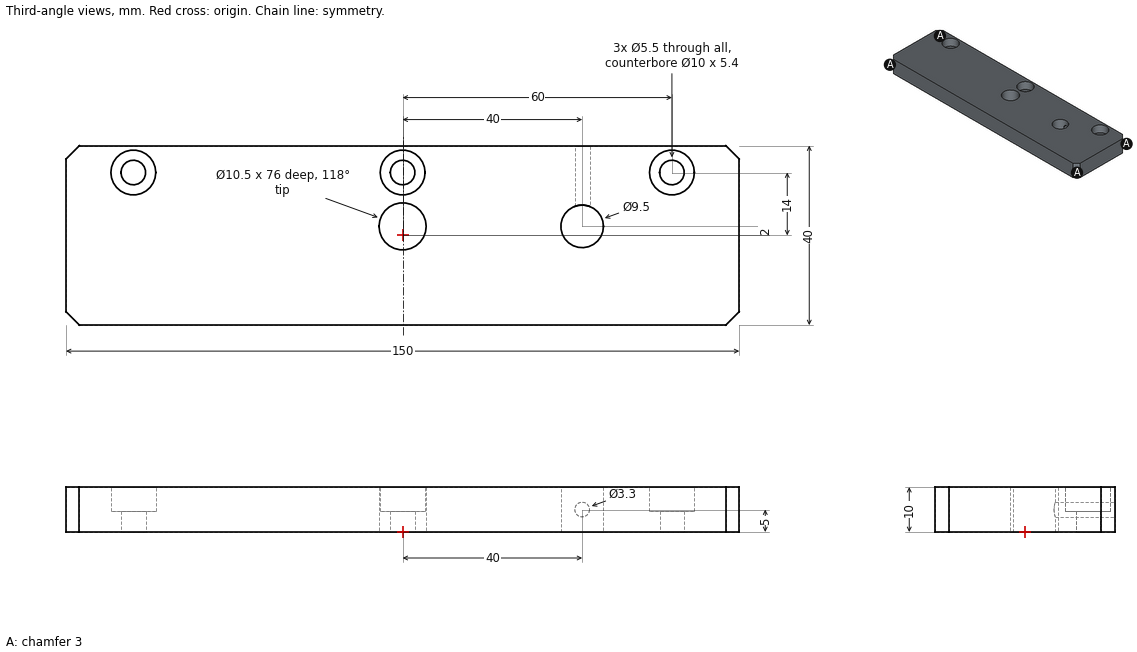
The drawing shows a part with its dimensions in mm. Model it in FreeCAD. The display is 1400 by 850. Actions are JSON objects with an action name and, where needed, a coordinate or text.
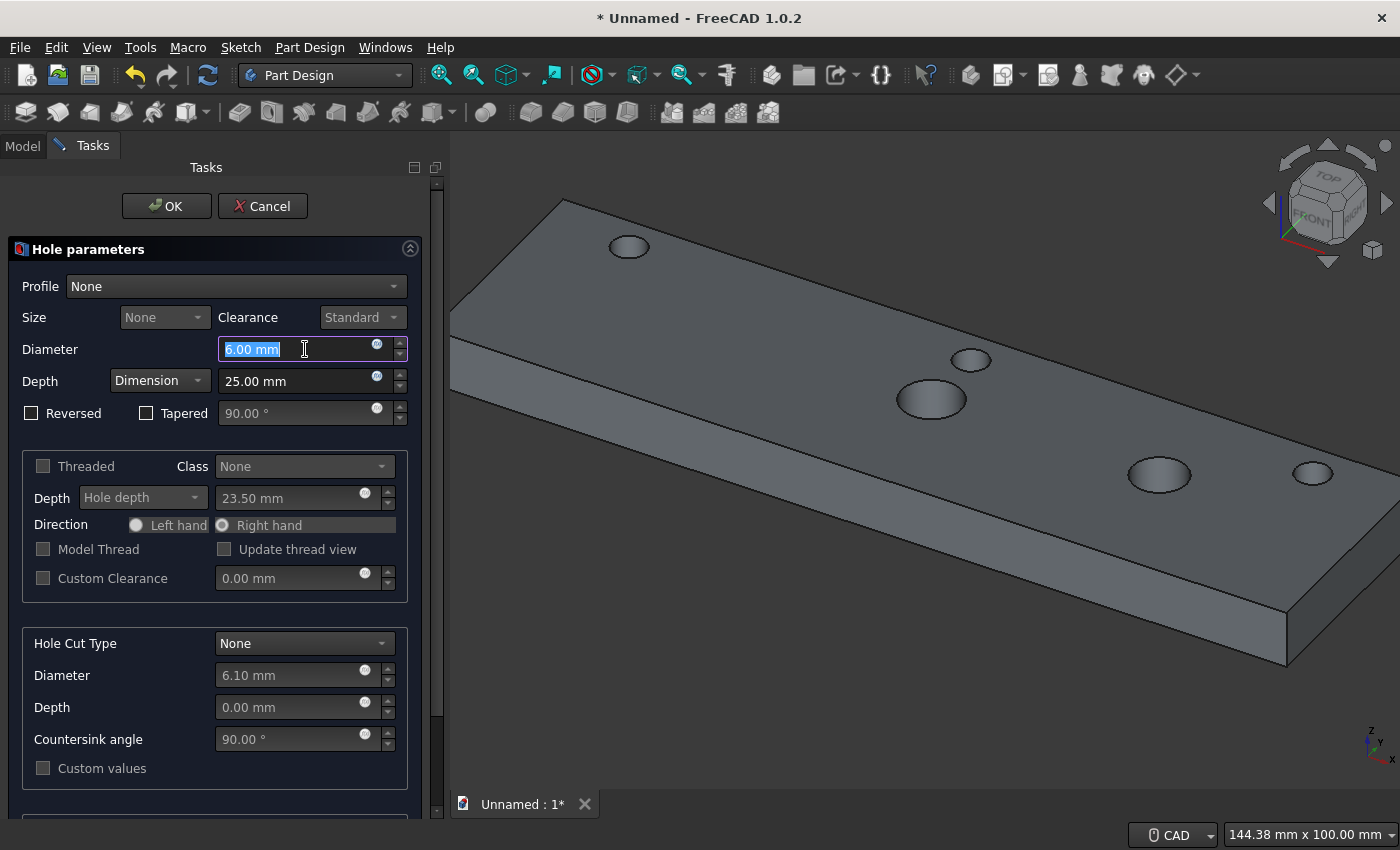
{"action": "type", "text": "5.5"}
{"action": "key", "text": "Tab"}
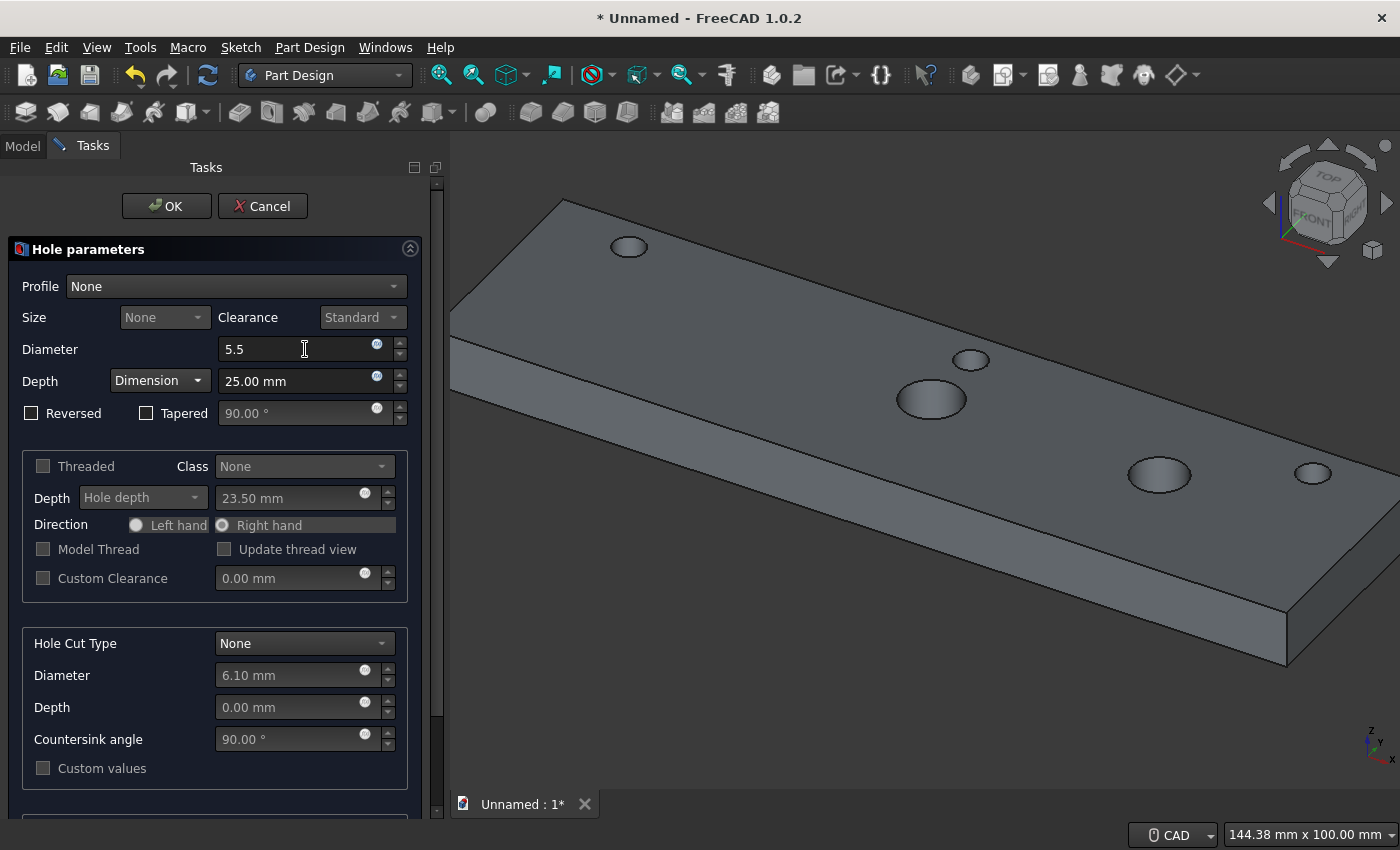
{"action": "left_click", "coordinate": [161, 380]}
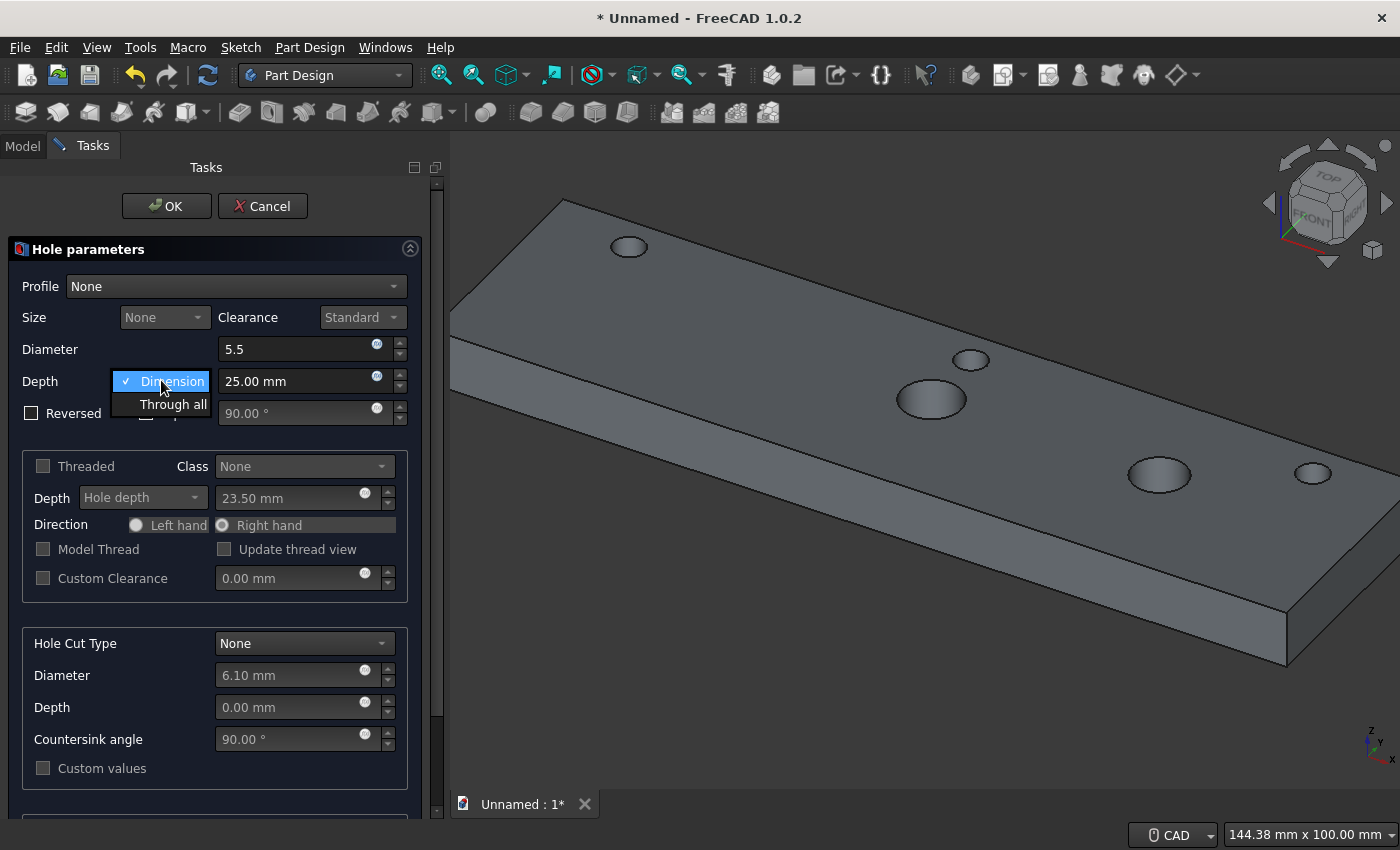
{"action": "left_click", "coordinate": [160, 404]}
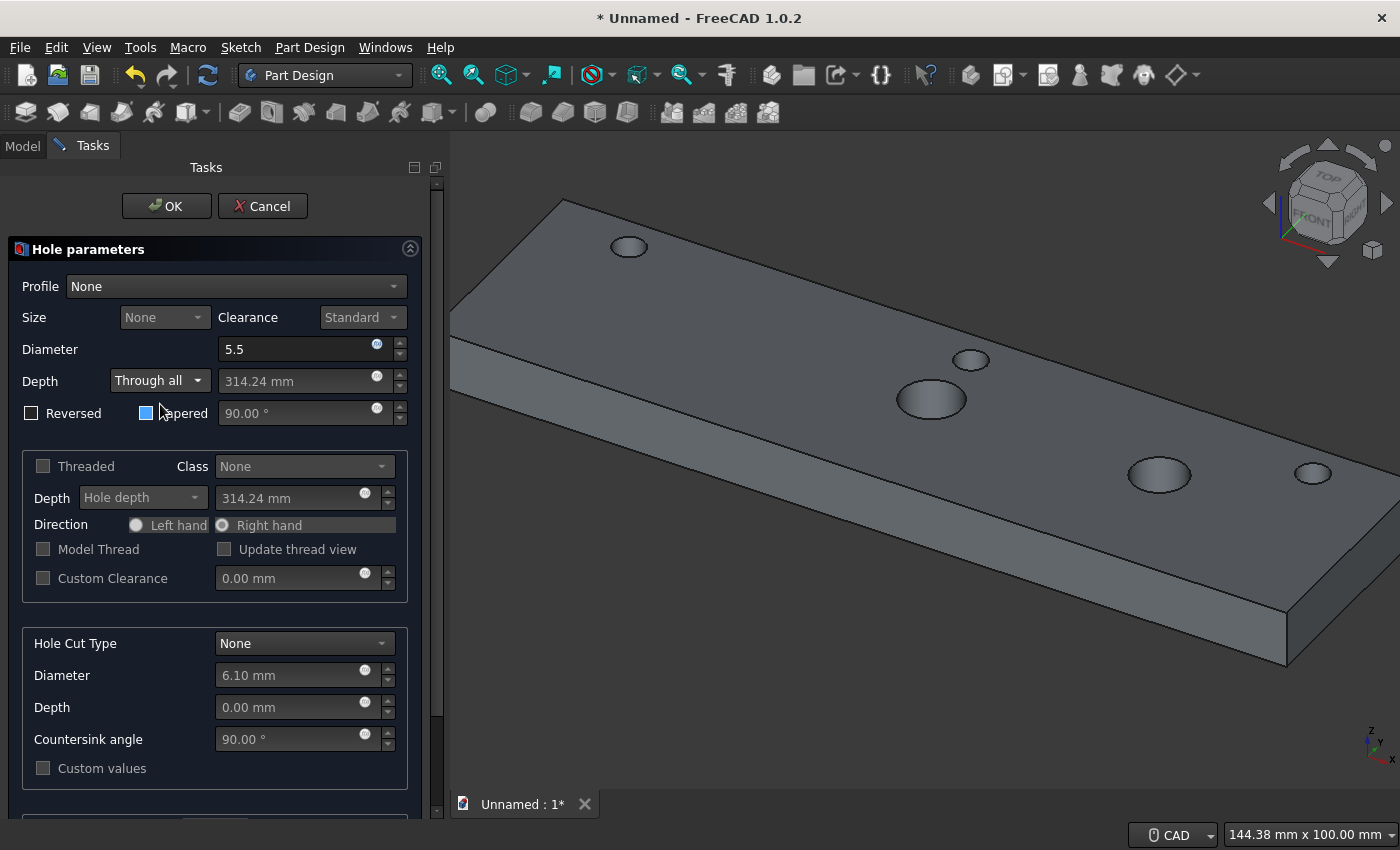
{"action": "left_click", "coordinate": [306, 644]}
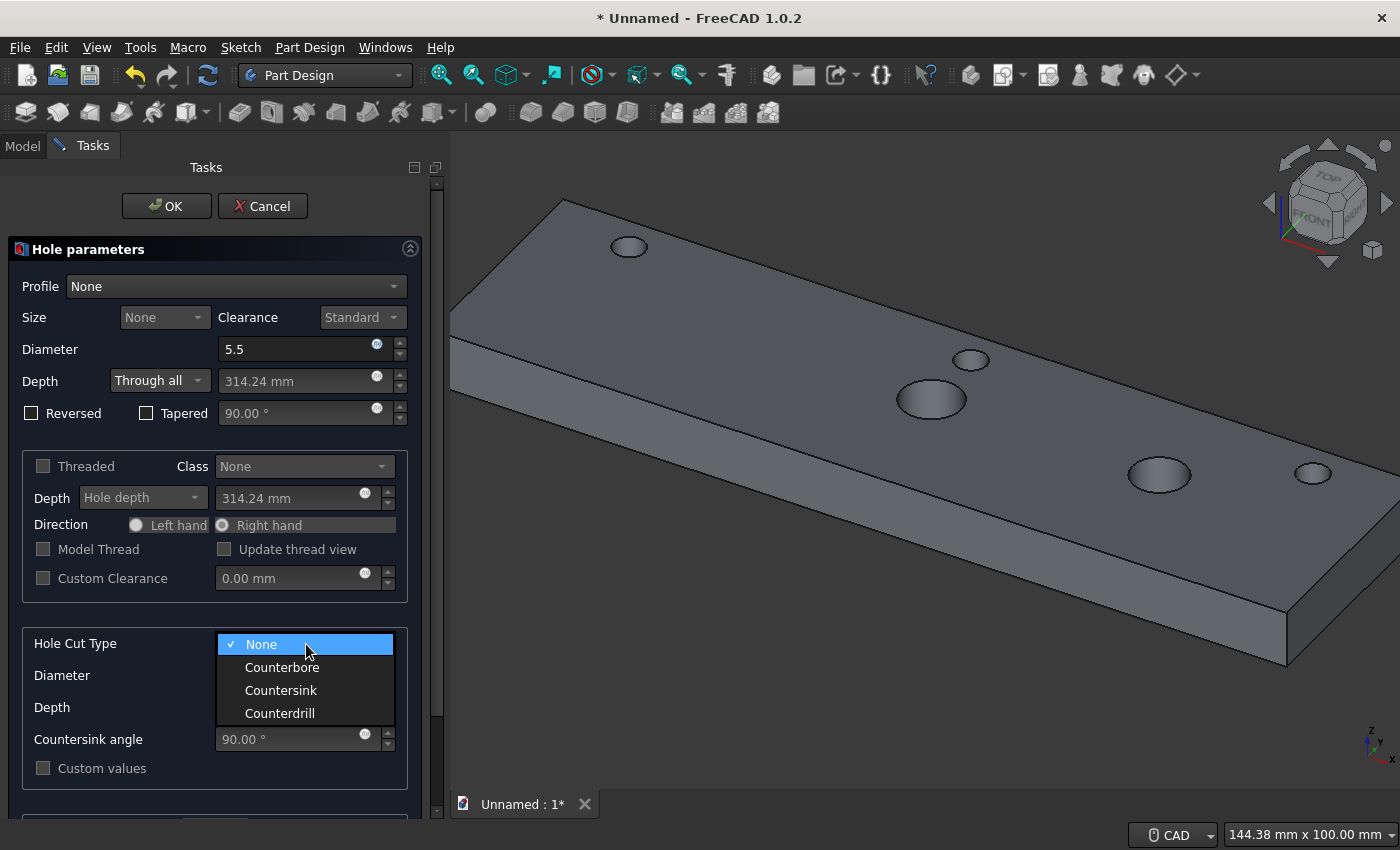
{"action": "left_click", "coordinate": [304, 668]}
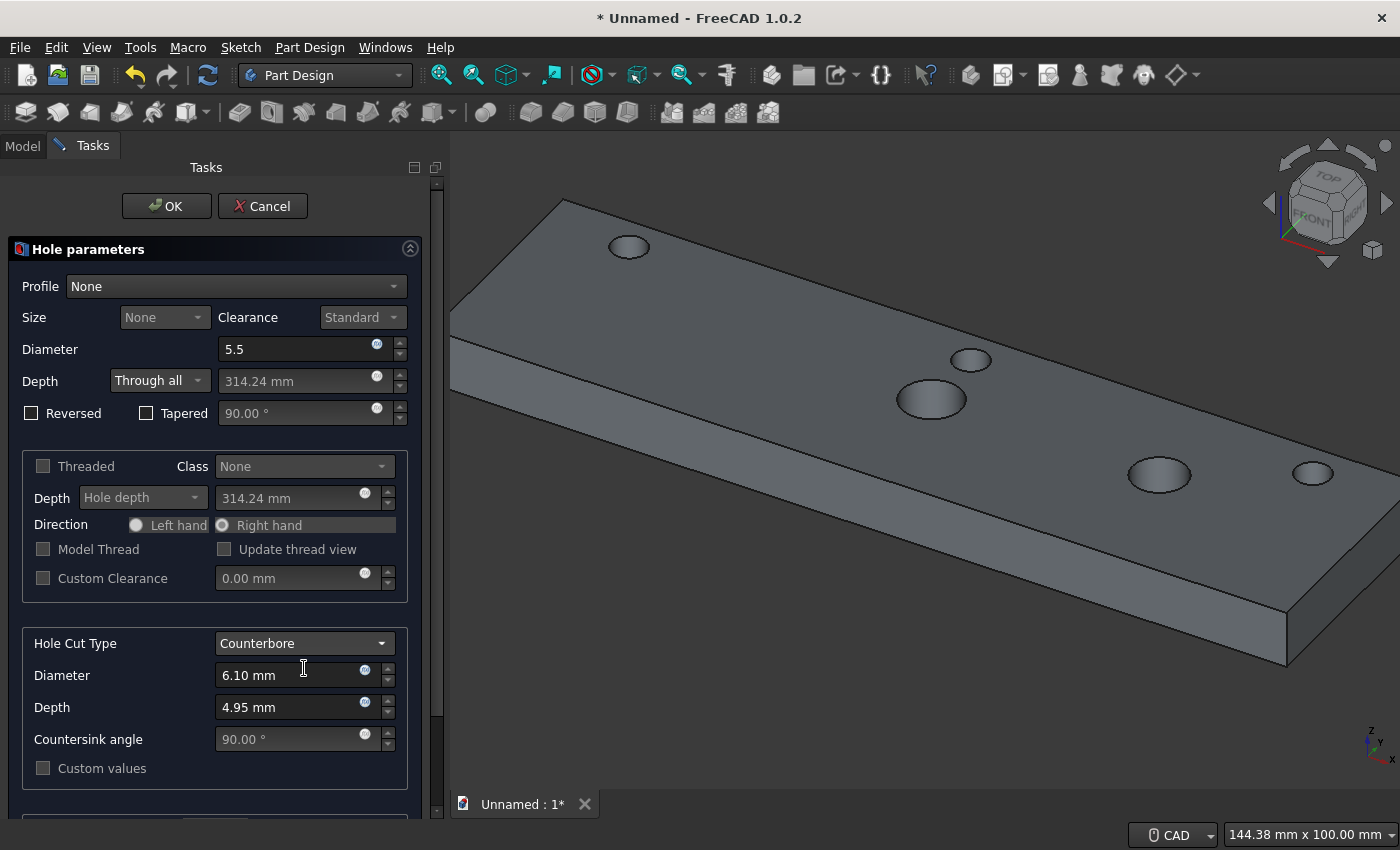
{"action": "triple_click", "coordinate": [298, 675]}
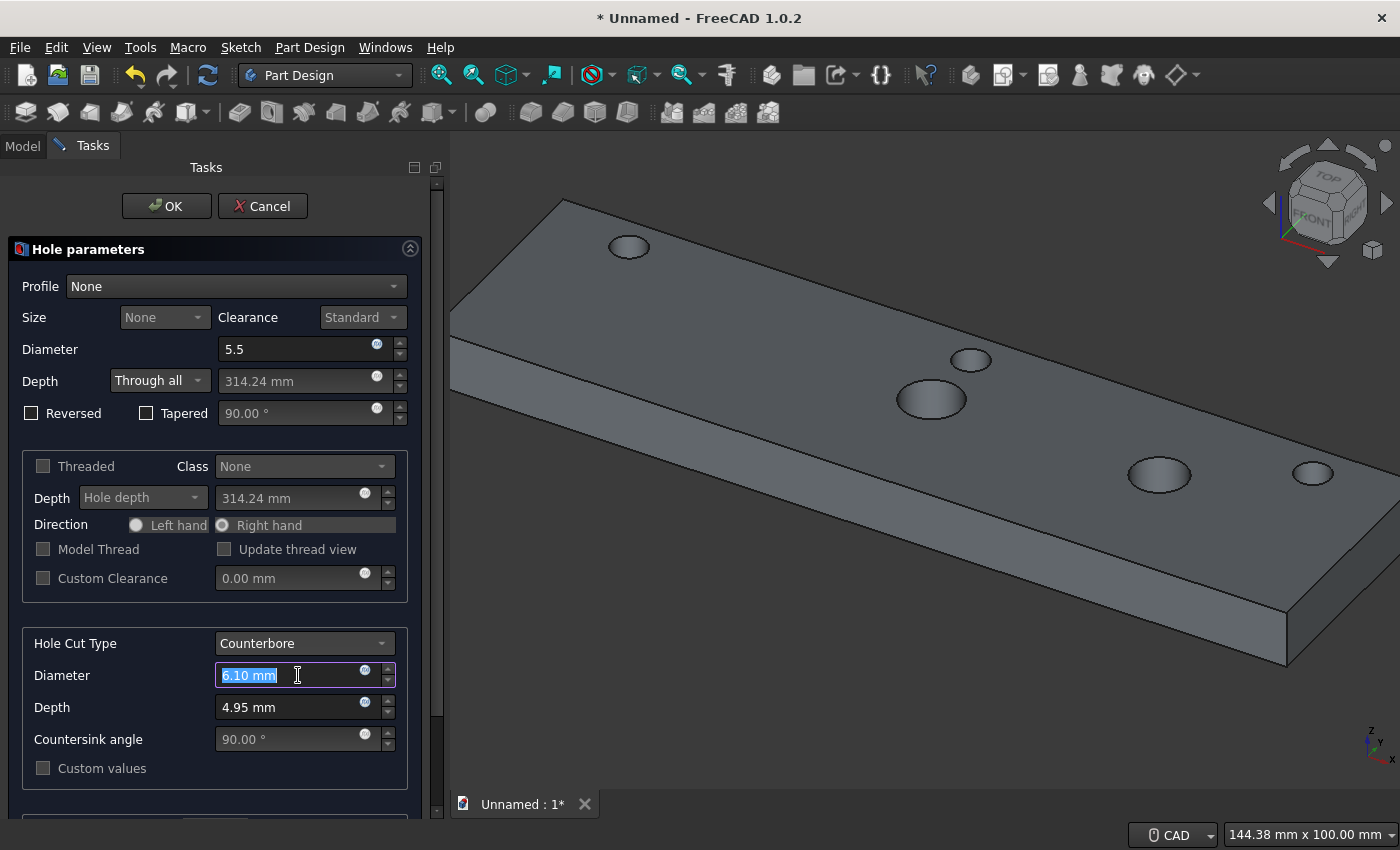
{"action": "type", "text": "10"}
{"action": "key", "text": "Tab"}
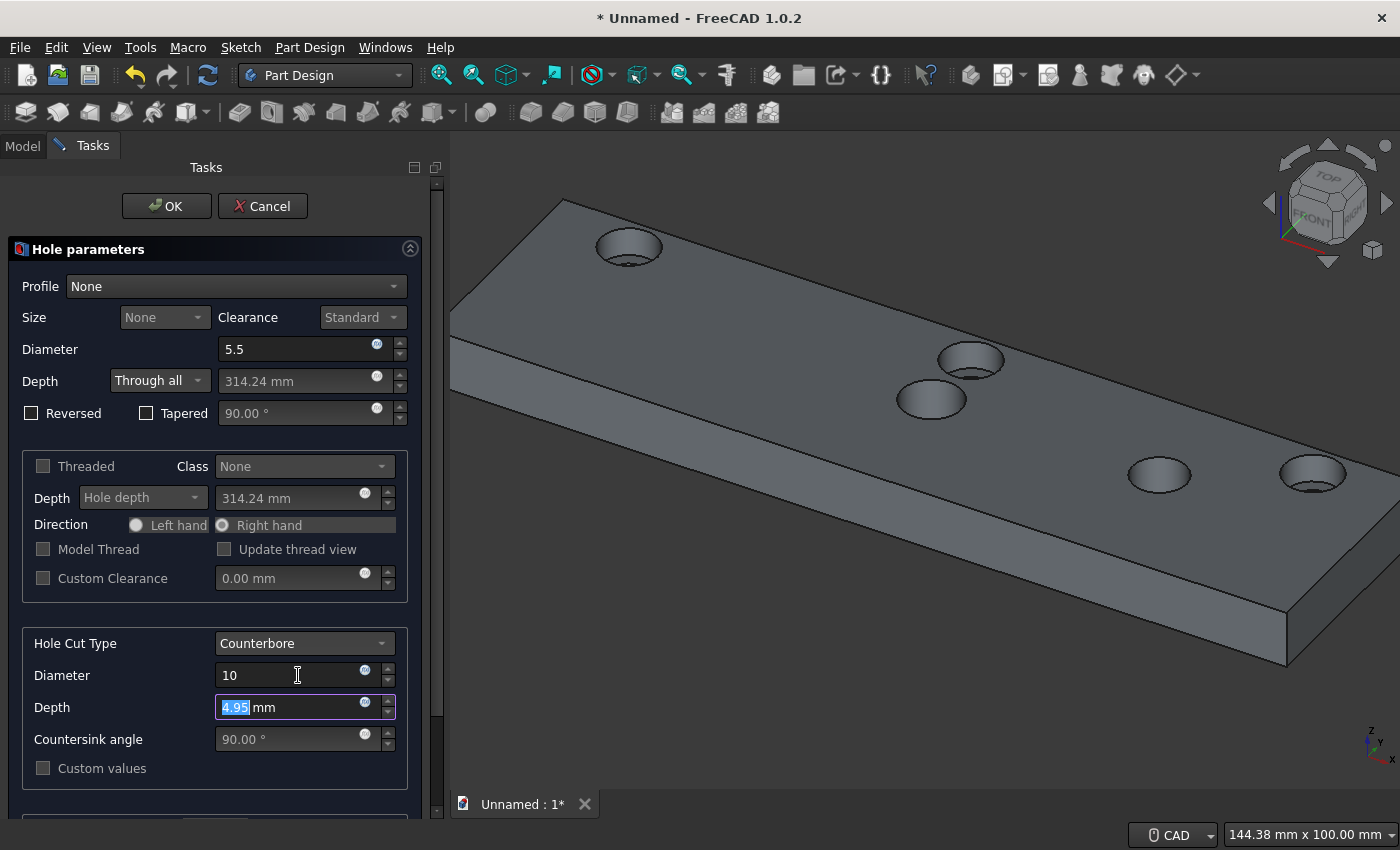
{"action": "type", "text": "5.4"}
{"action": "key", "text": "Tab"}